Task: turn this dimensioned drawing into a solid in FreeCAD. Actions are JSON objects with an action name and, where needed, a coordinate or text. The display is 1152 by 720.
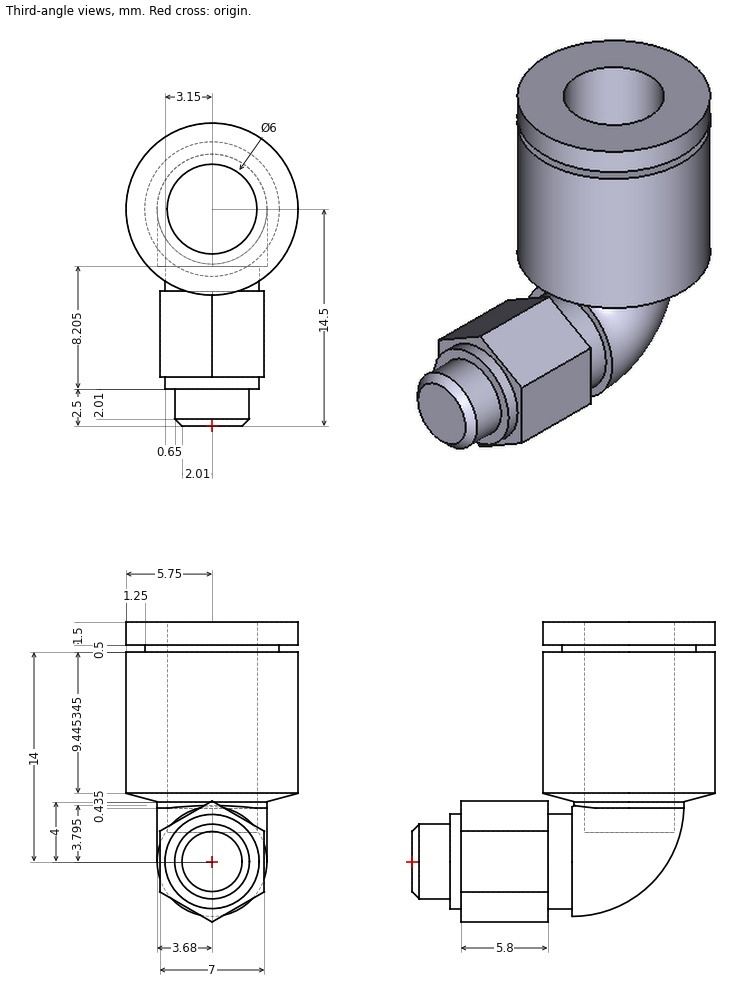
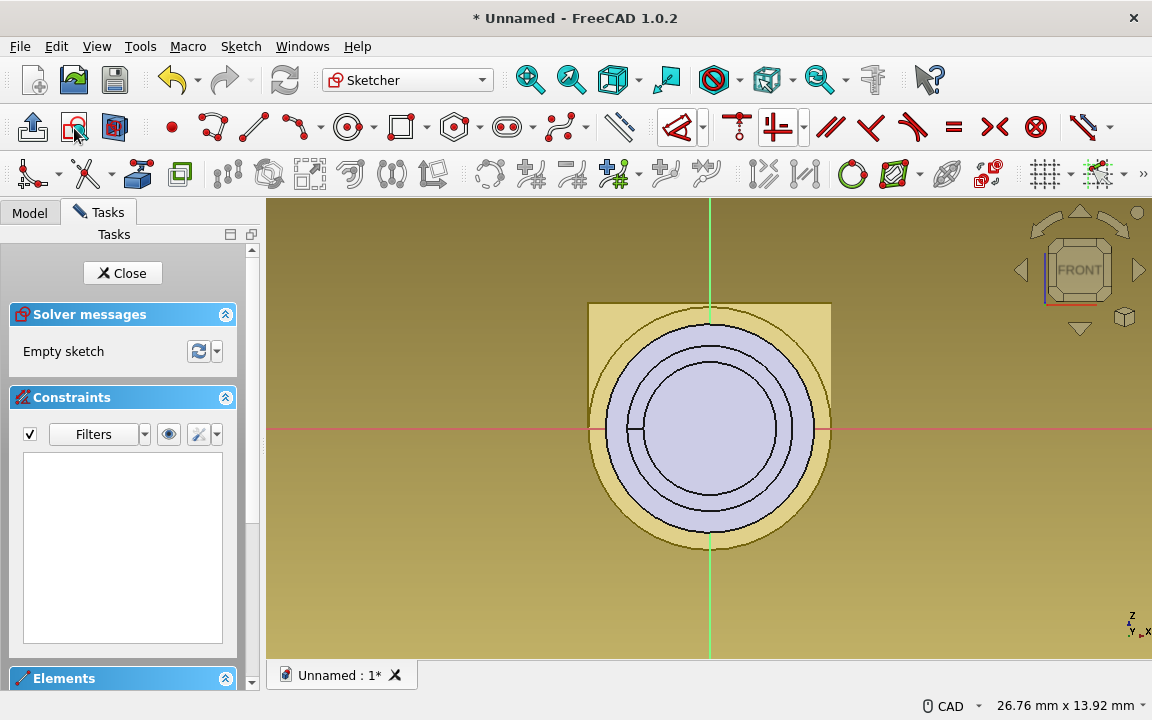
{"action": "left_click", "coordinate": [115, 128]}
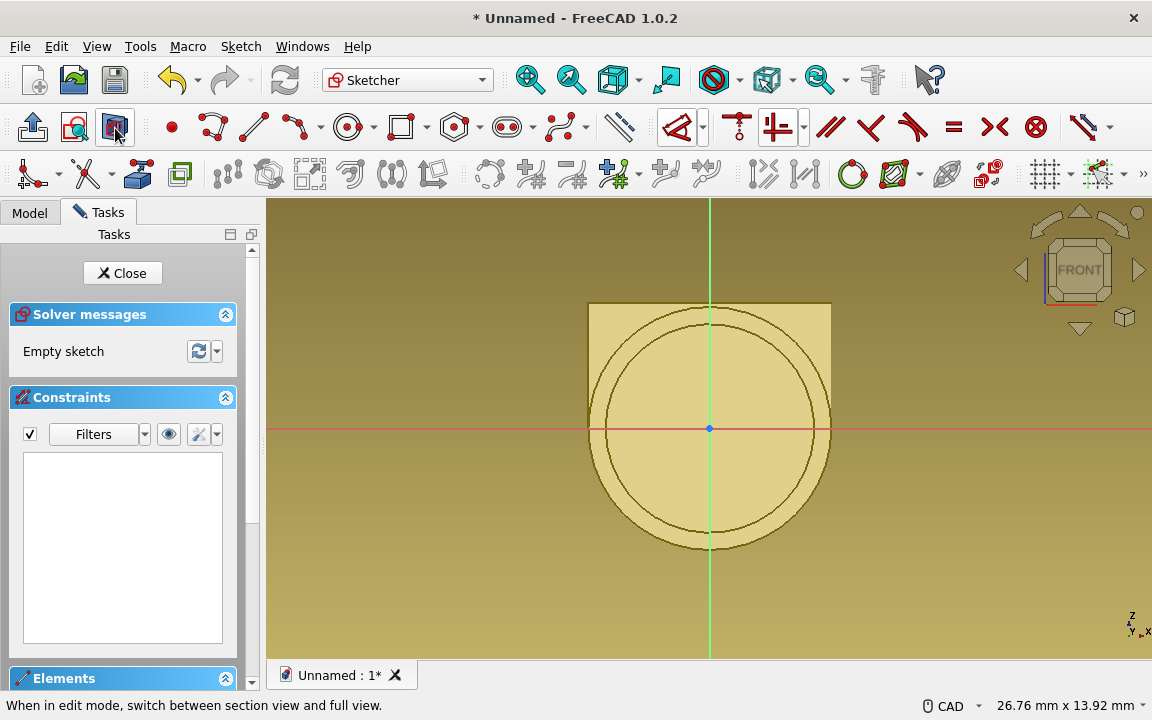
{"action": "left_click", "coordinate": [454, 128]}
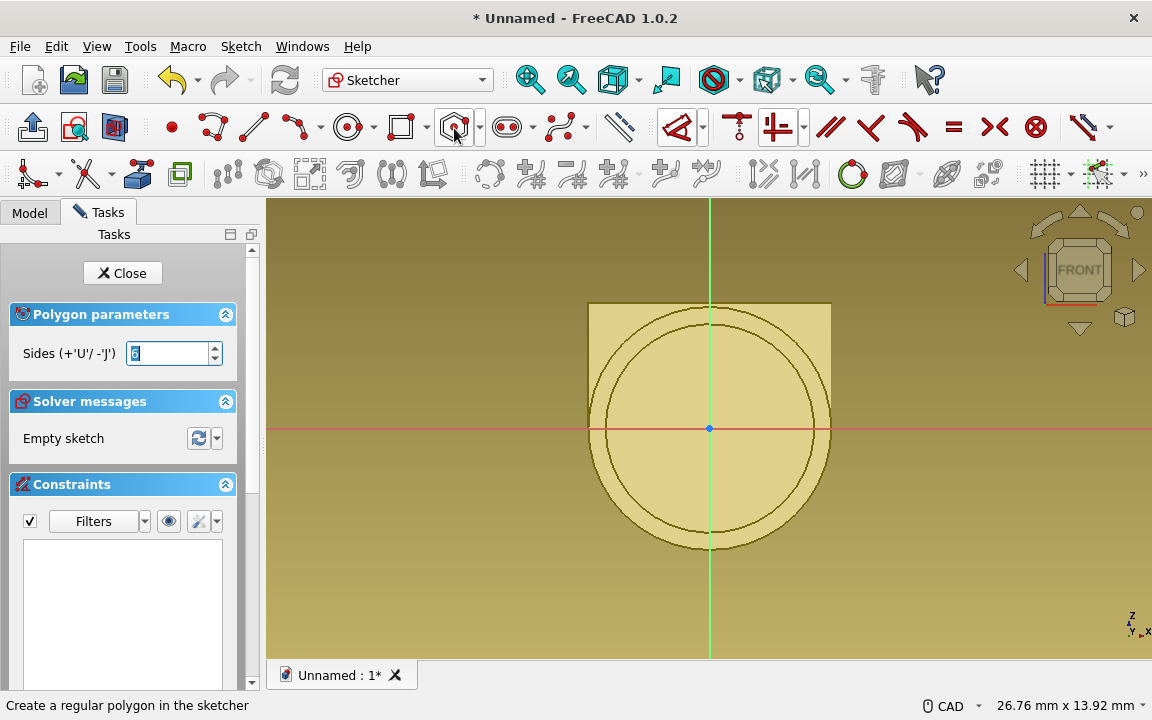
{"action": "left_click", "coordinate": [710, 428]}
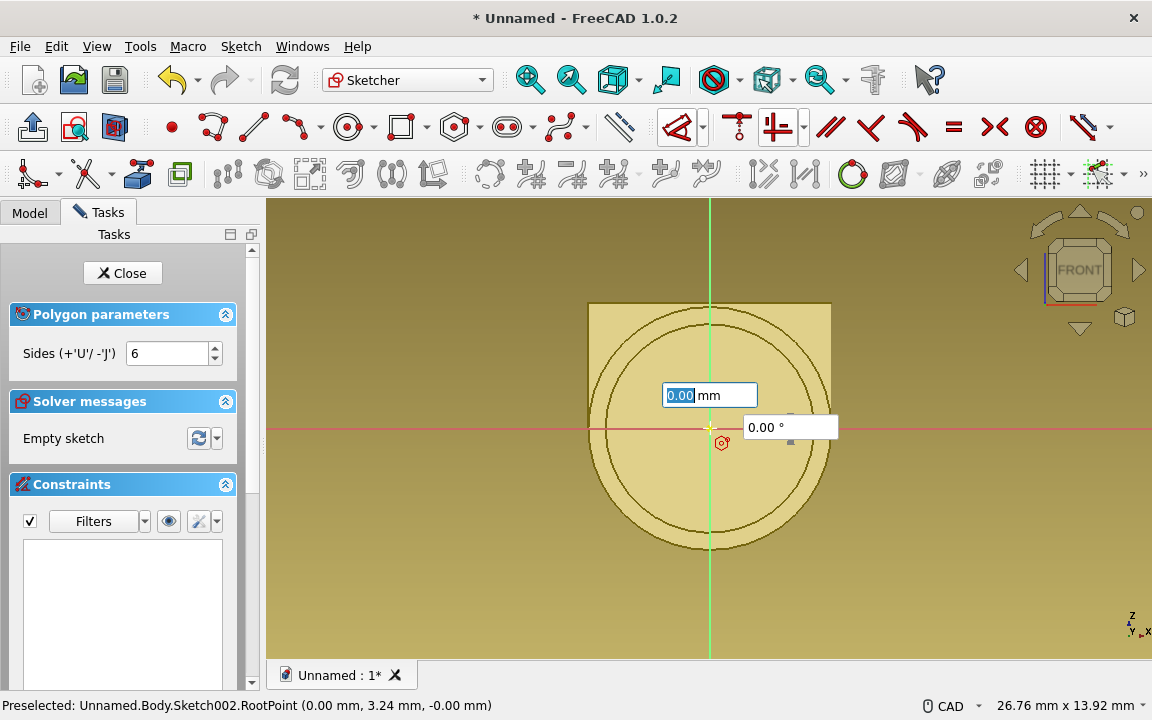
{"action": "left_click", "coordinate": [710, 295]}
{"action": "right_click", "coordinate": [710, 295]}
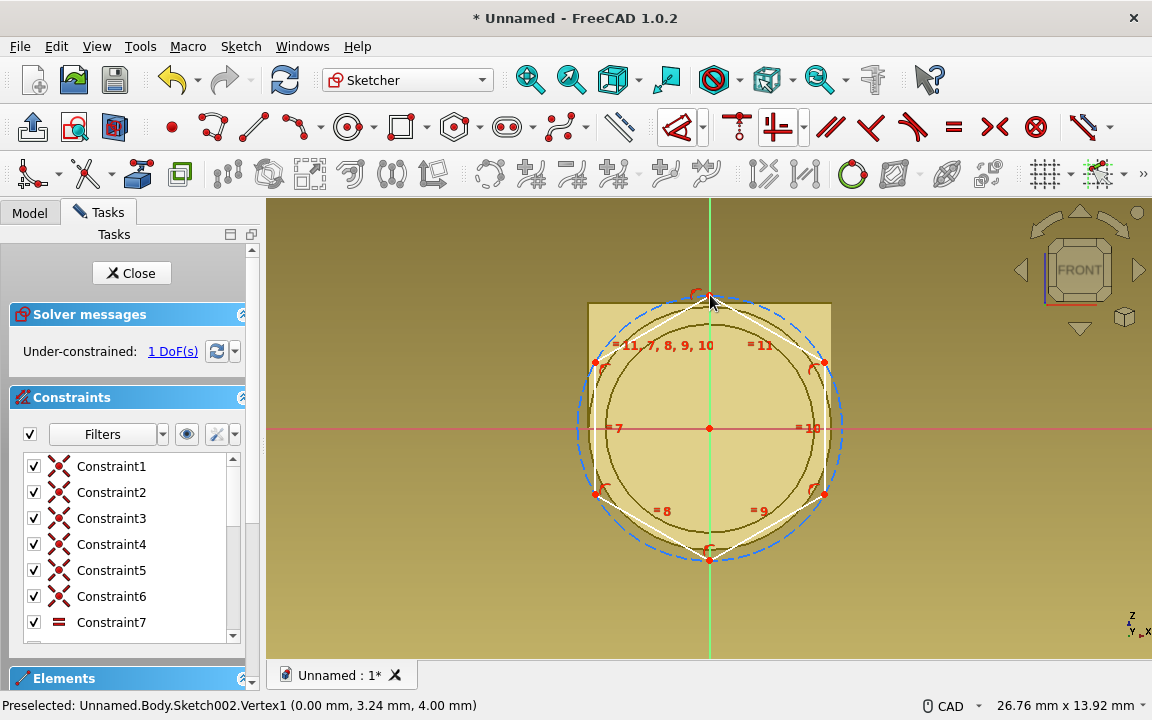
{"action": "left_click", "coordinate": [595, 362]}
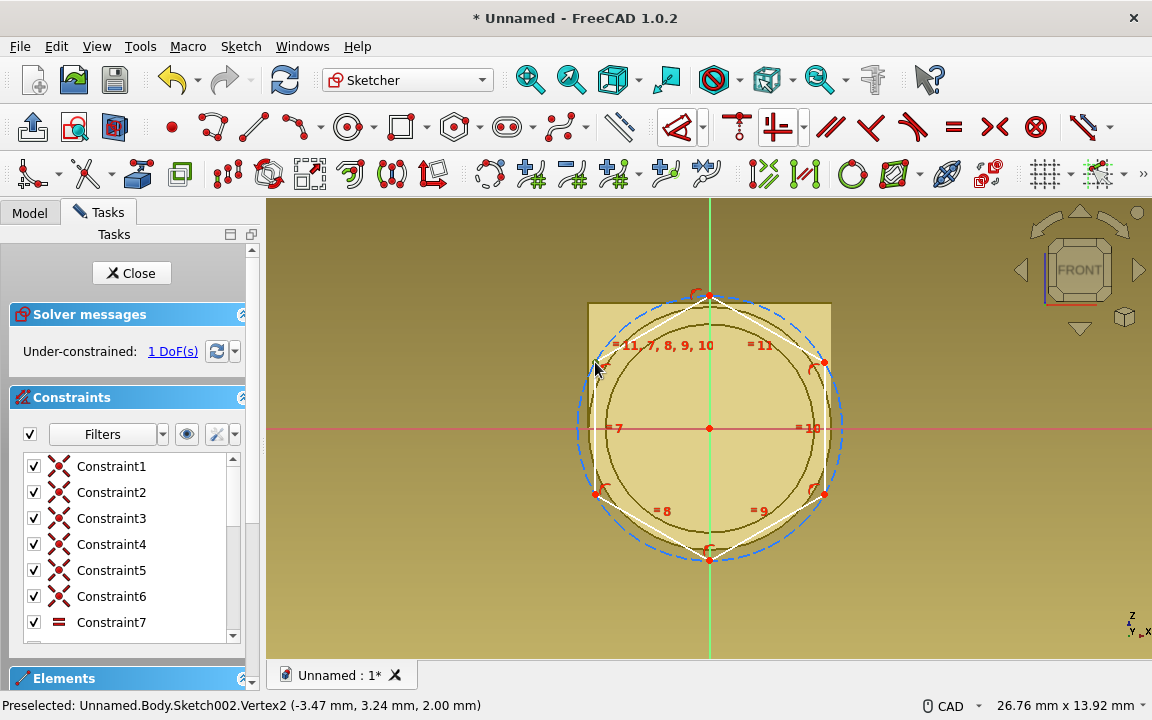
{"action": "left_click", "coordinate": [825, 495]}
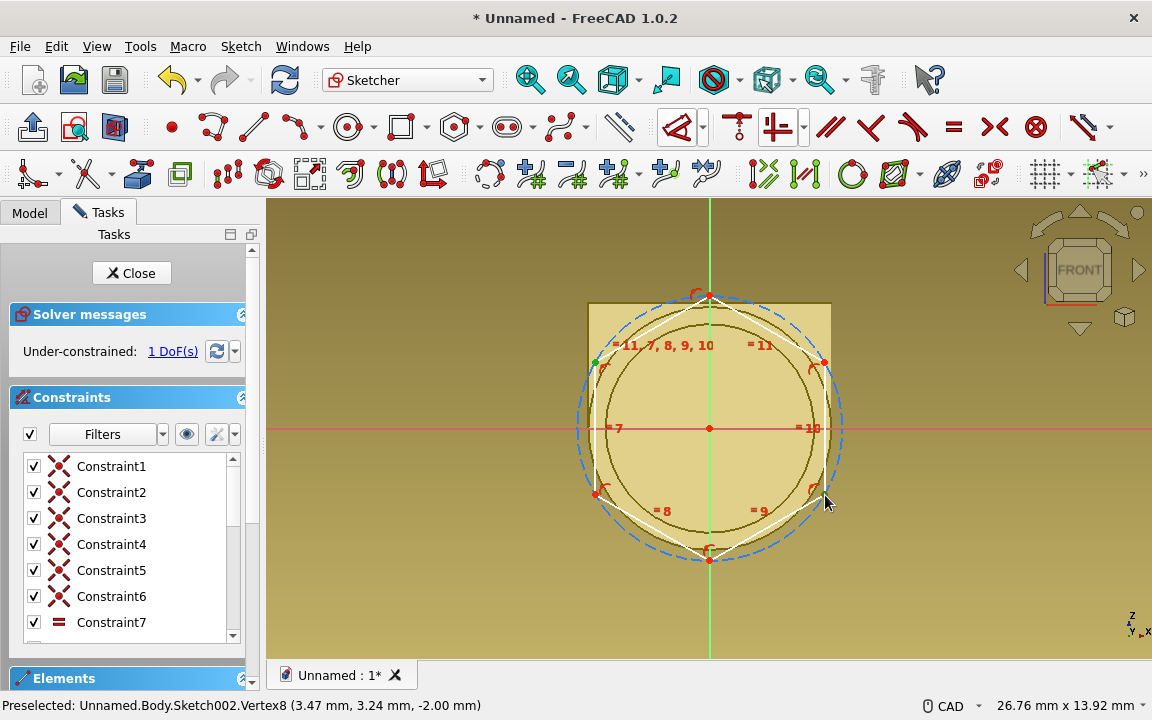
{"action": "key", "text": "l"}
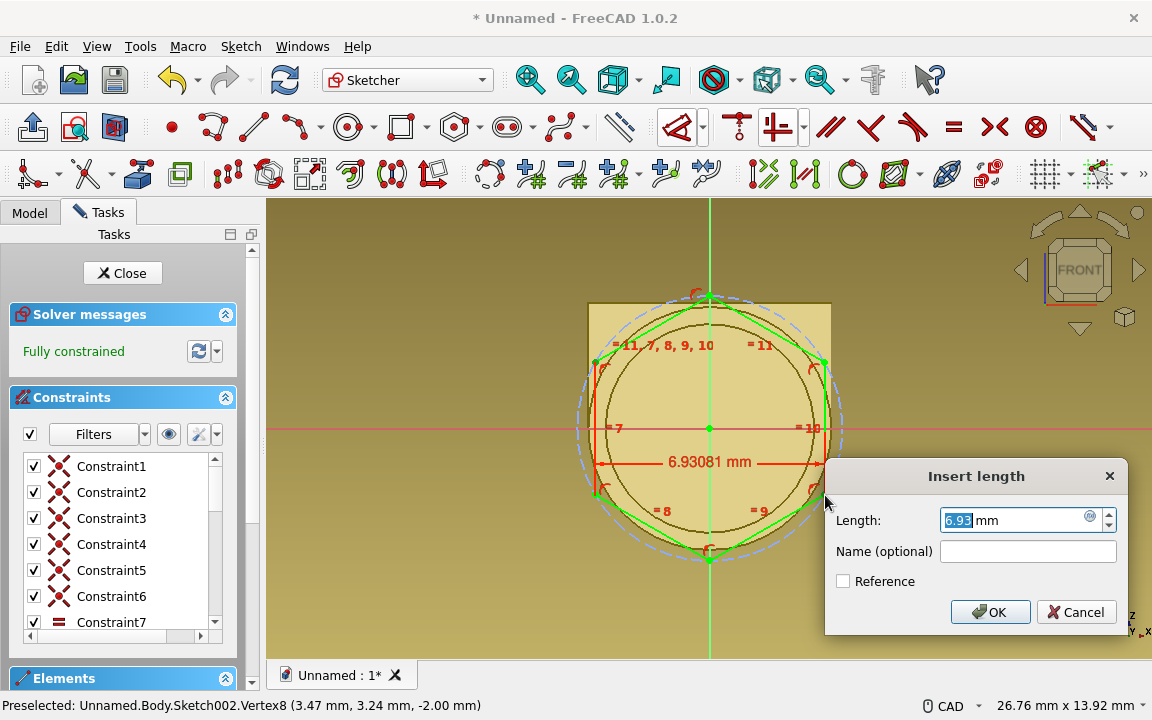
{"action": "type", "text": "7"}
{"action": "key", "text": "Return"}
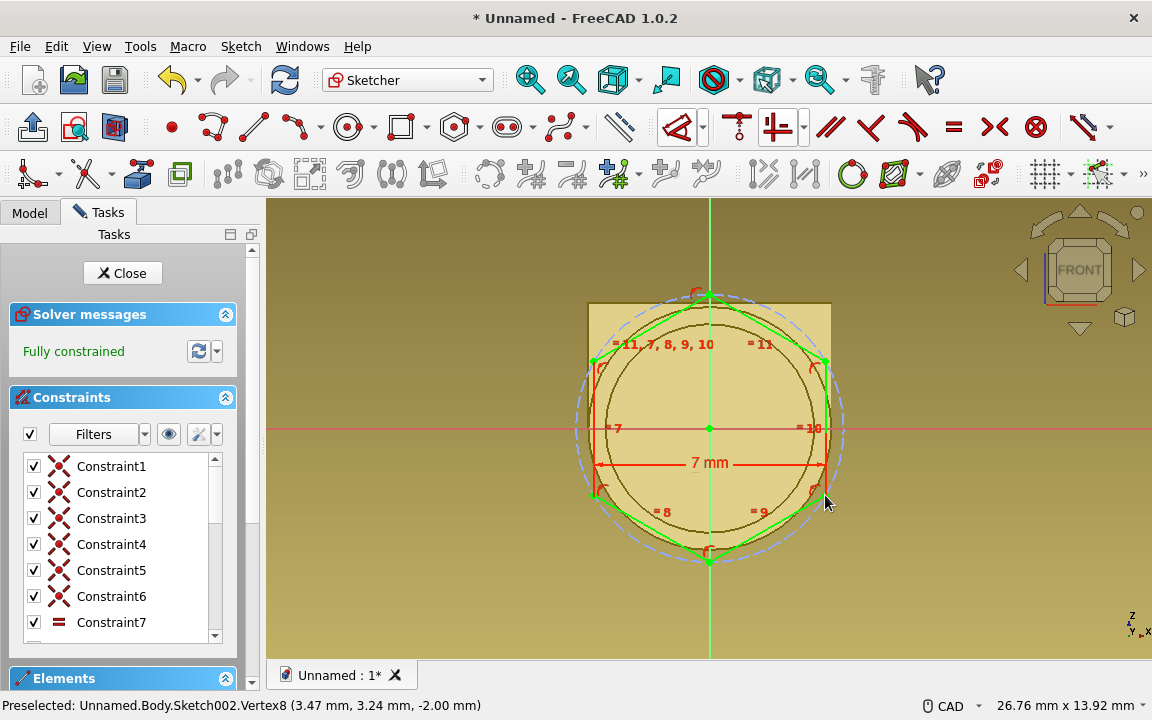
{"action": "left_click", "coordinate": [123, 273]}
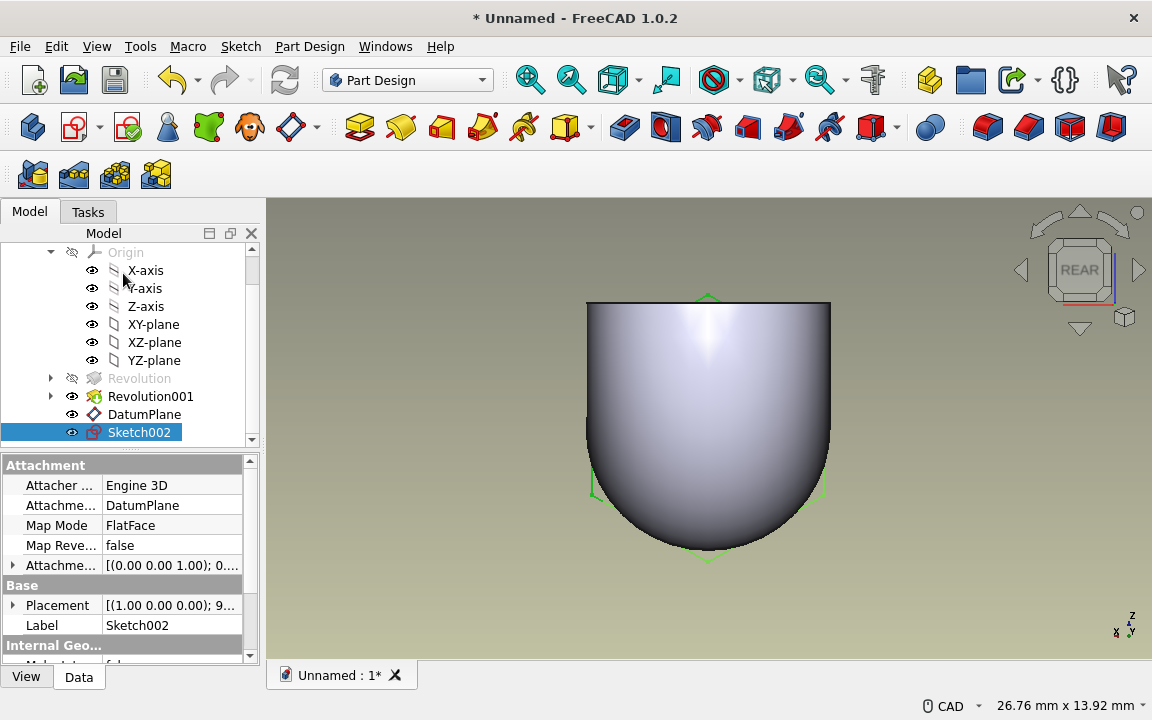
{"action": "left_click", "coordinate": [360, 128]}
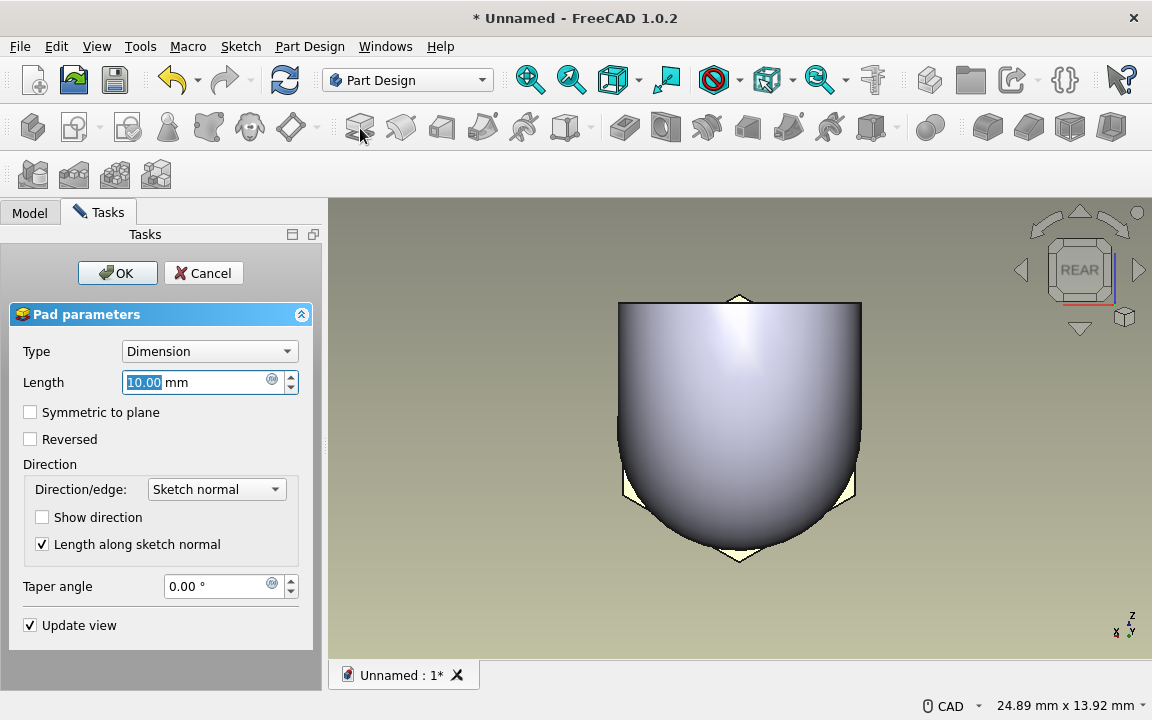
{"action": "type", "text": "5.8"}
{"action": "key", "text": "Tab"}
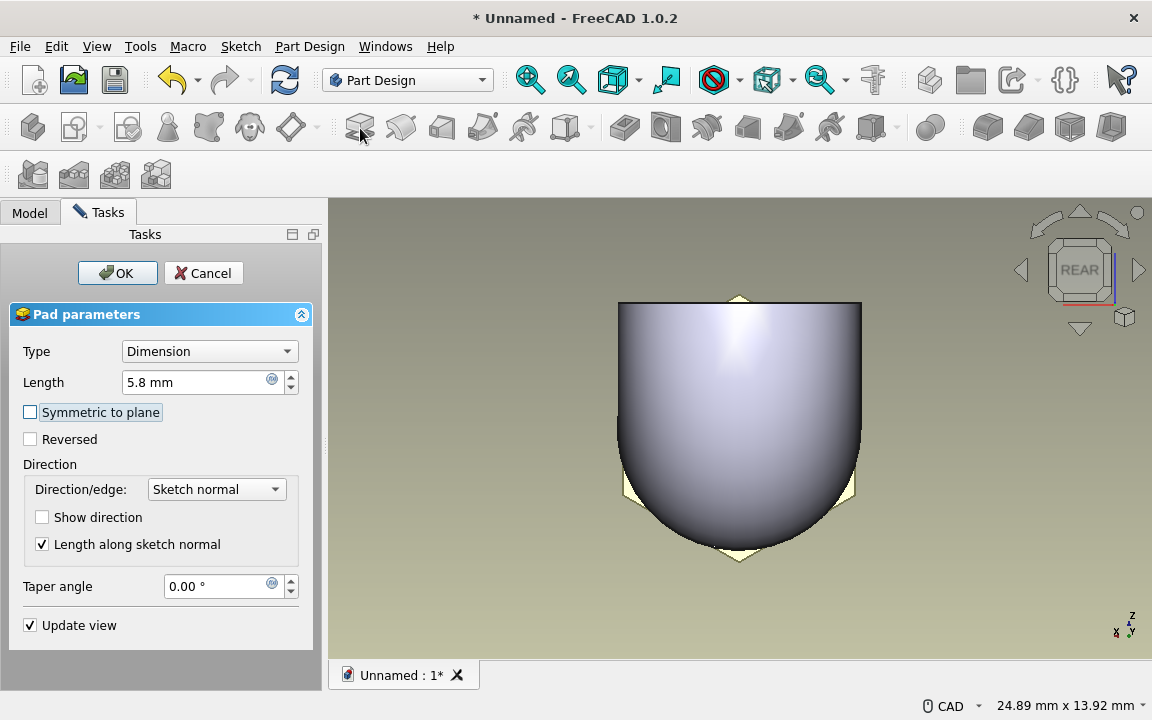
{"action": "left_click", "coordinate": [31, 439]}